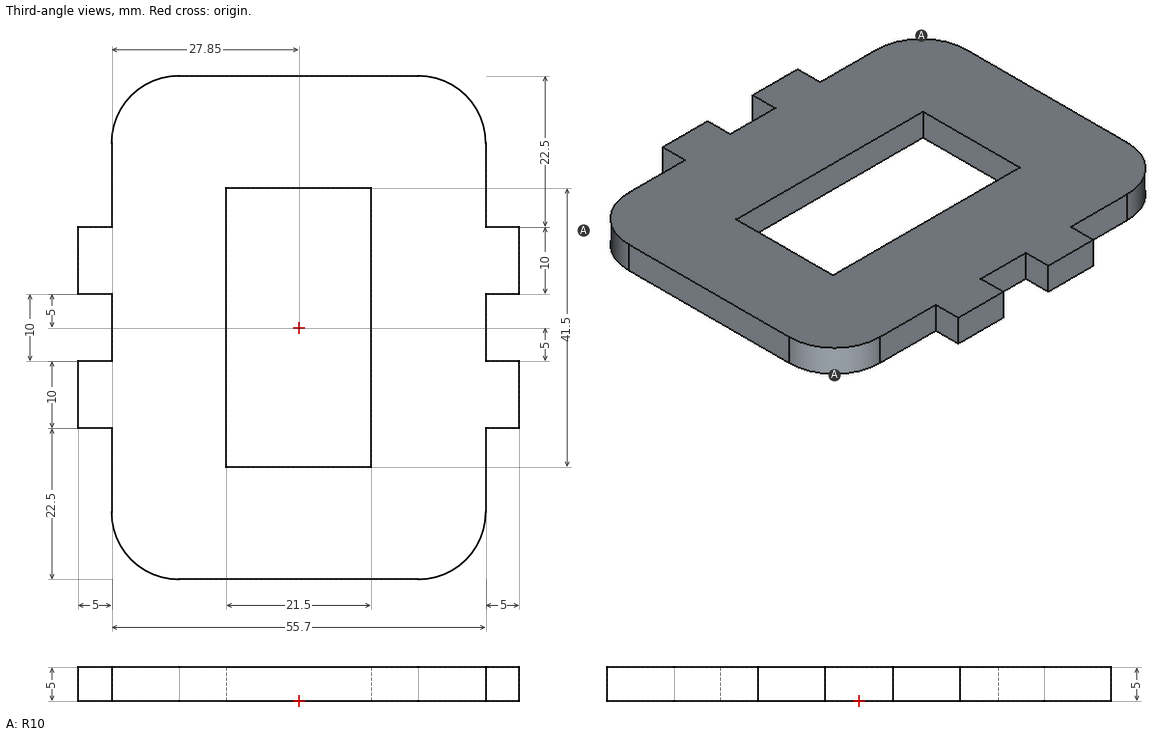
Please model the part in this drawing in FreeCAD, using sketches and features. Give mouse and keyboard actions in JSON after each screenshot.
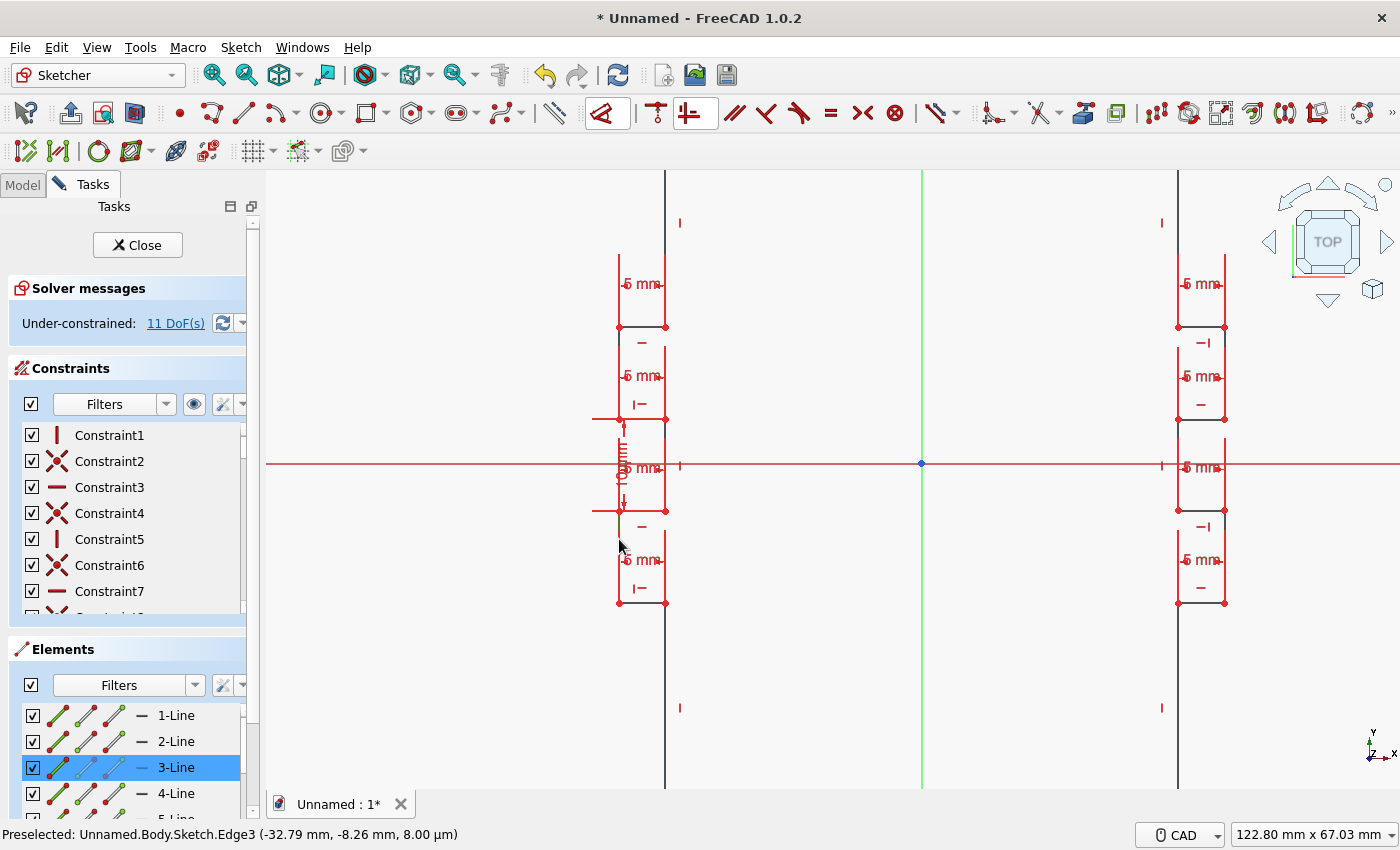
{"action": "key", "text": "i"}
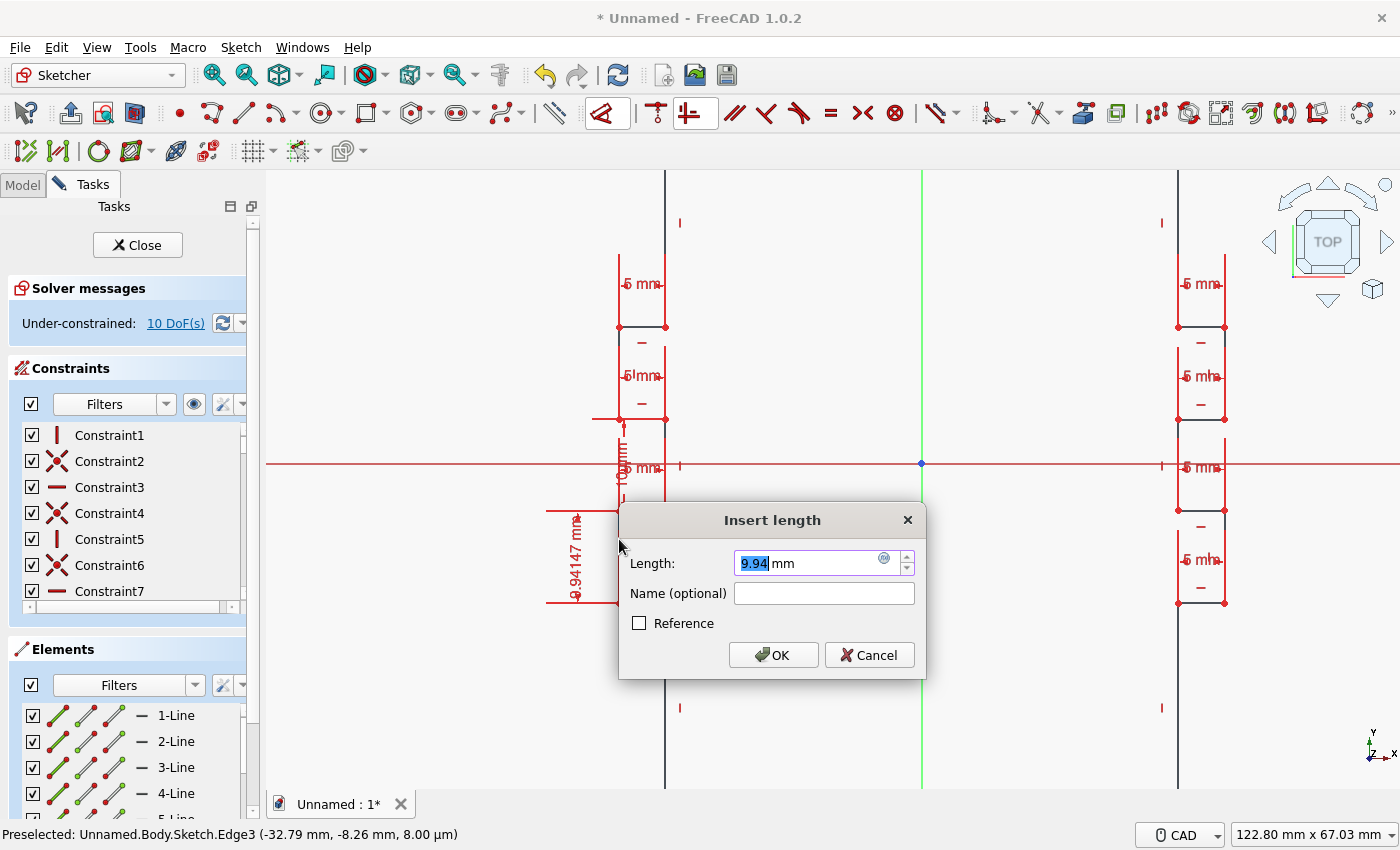
{"action": "type", "text": "10"}
{"action": "key", "text": "Return"}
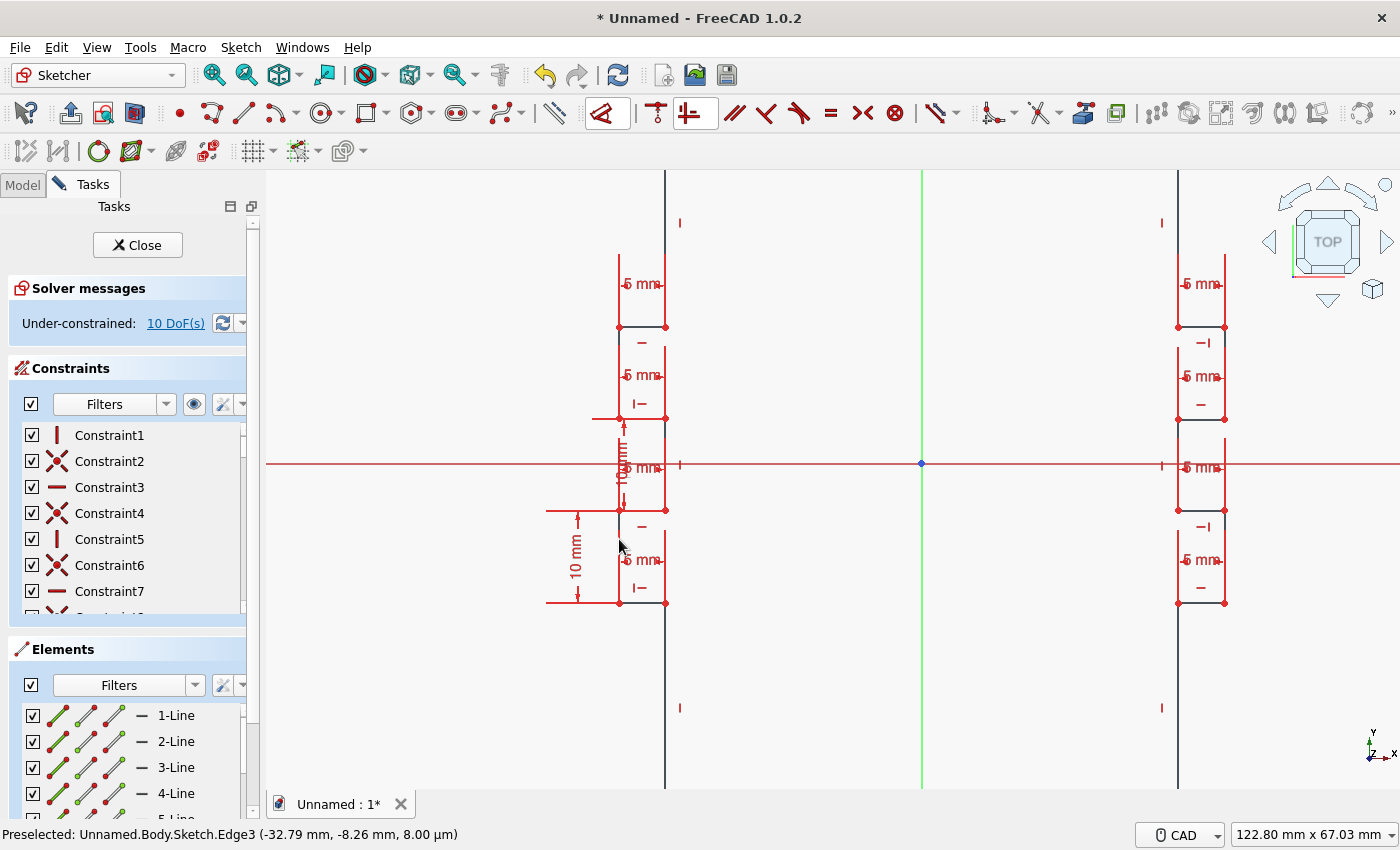
{"action": "left_click", "coordinate": [1225, 575]}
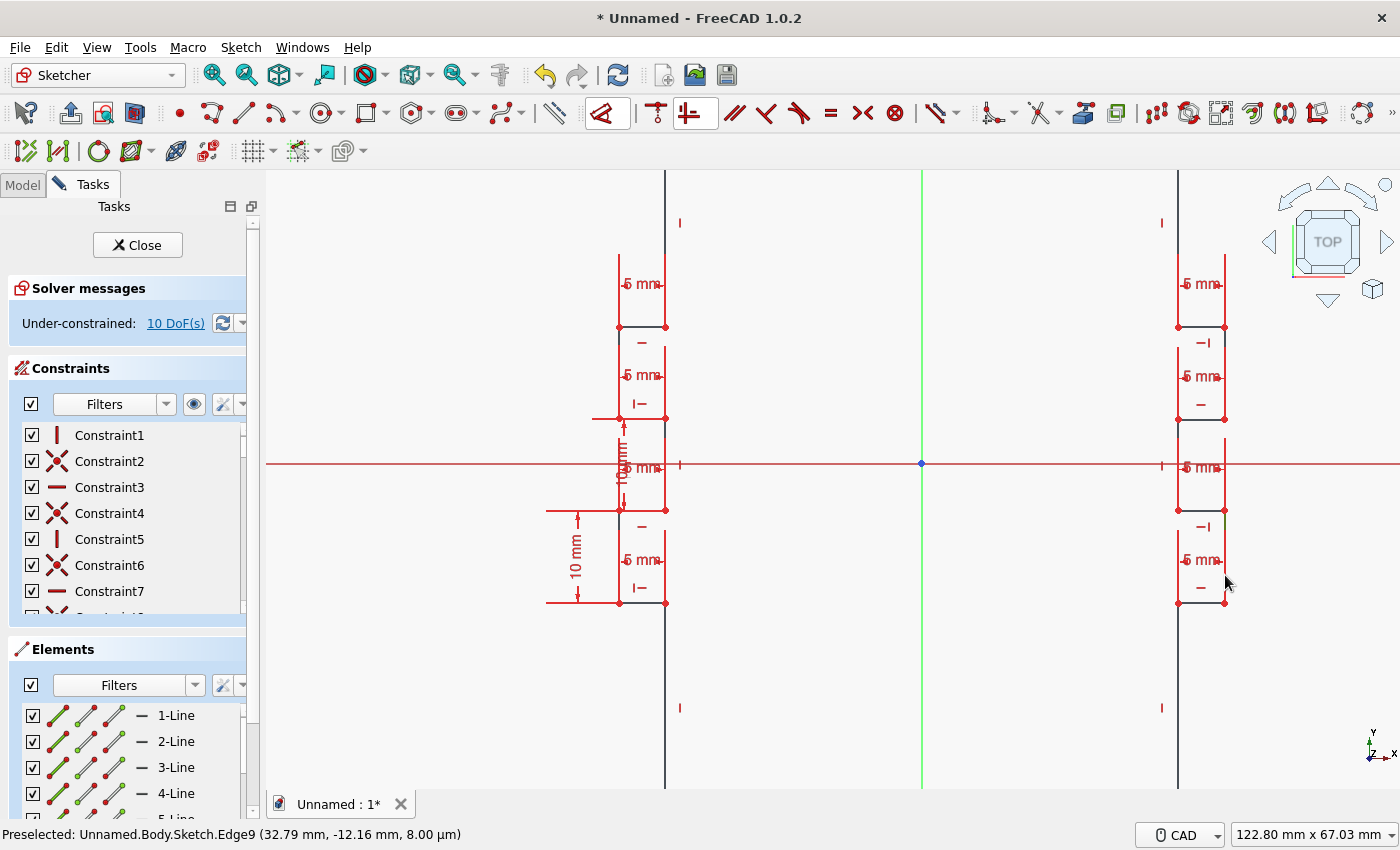
{"action": "key", "text": "i"}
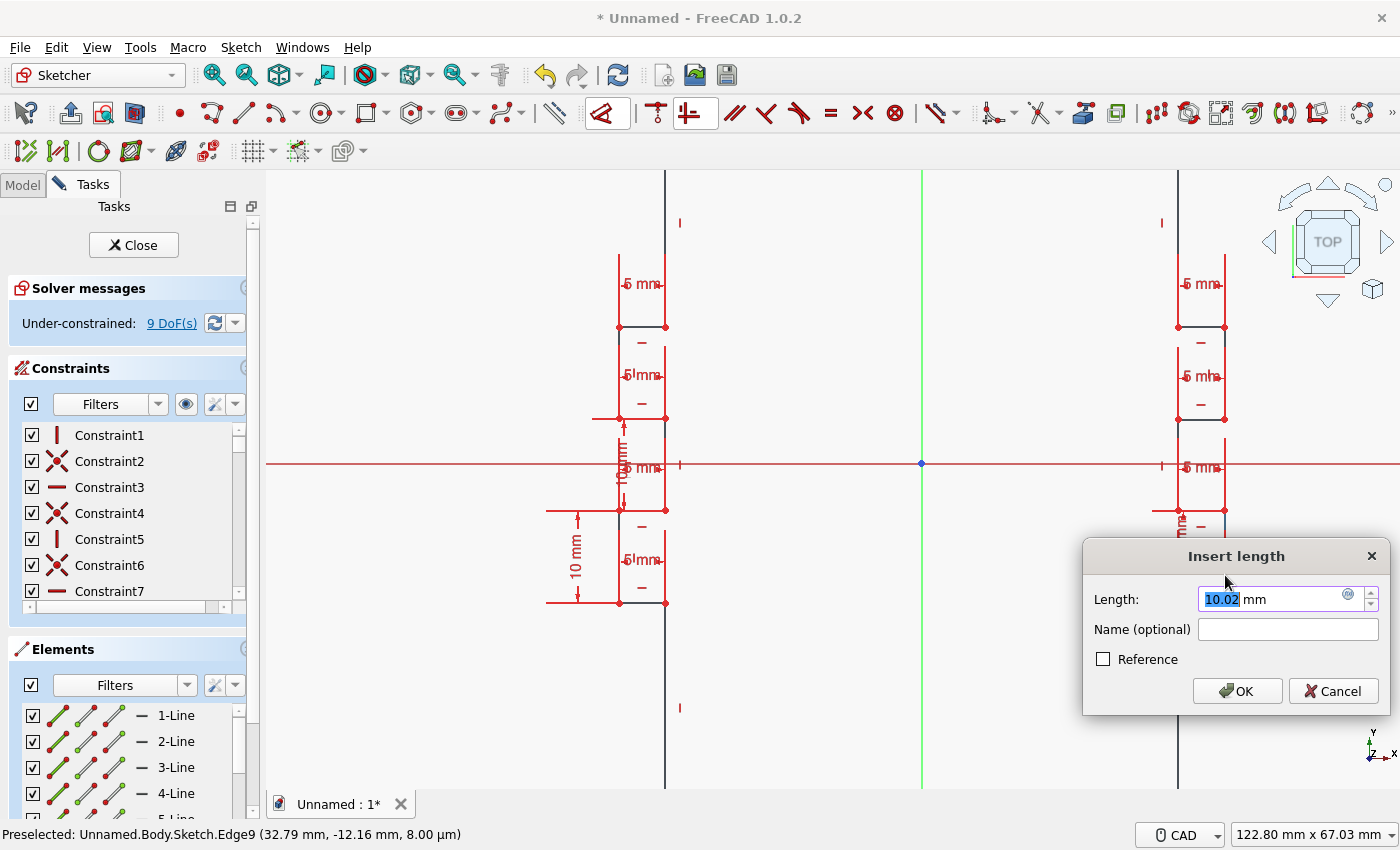
{"action": "type", "text": "10"}
{"action": "key", "text": "Return"}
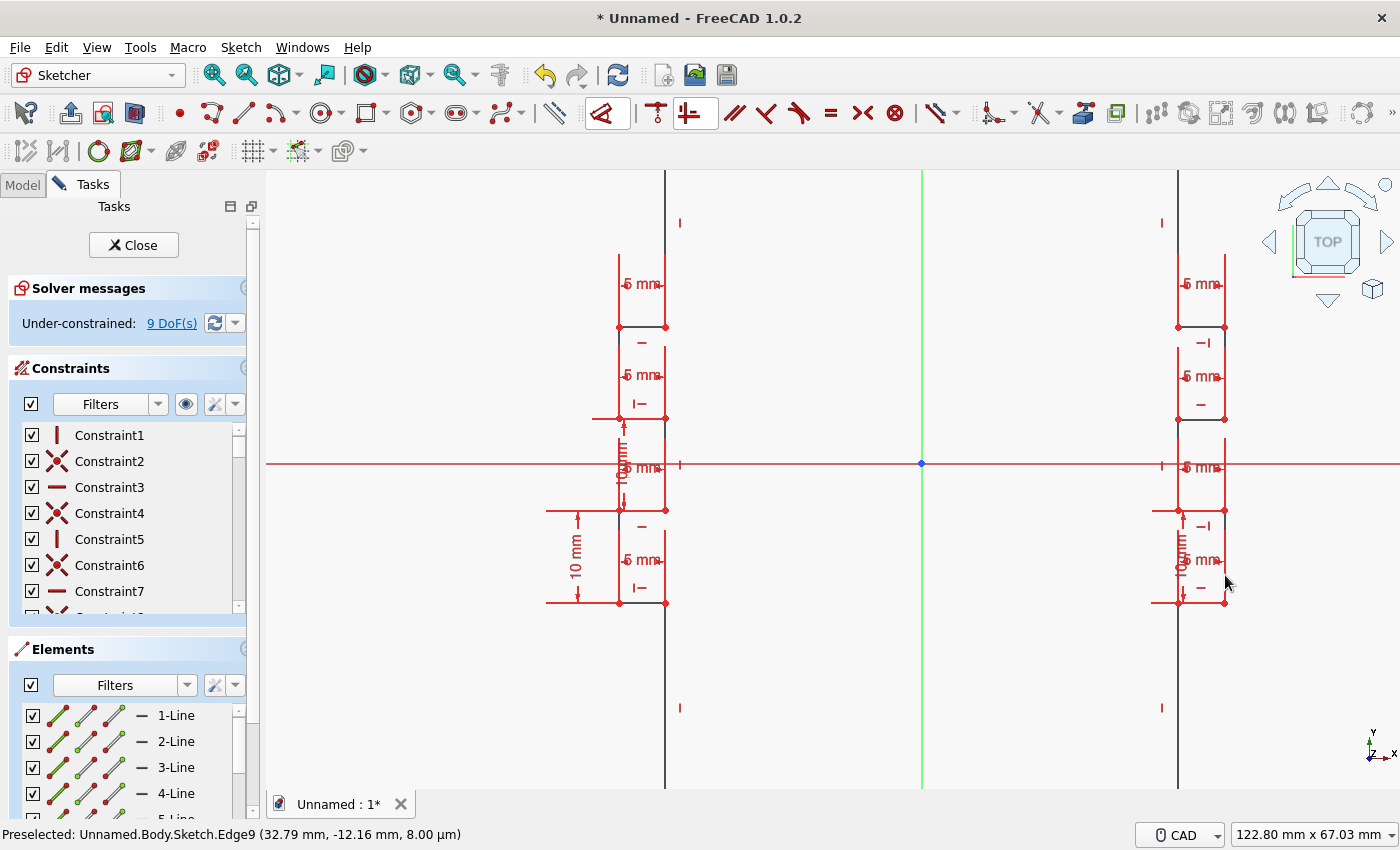
{"action": "left_click", "coordinate": [1178, 483]}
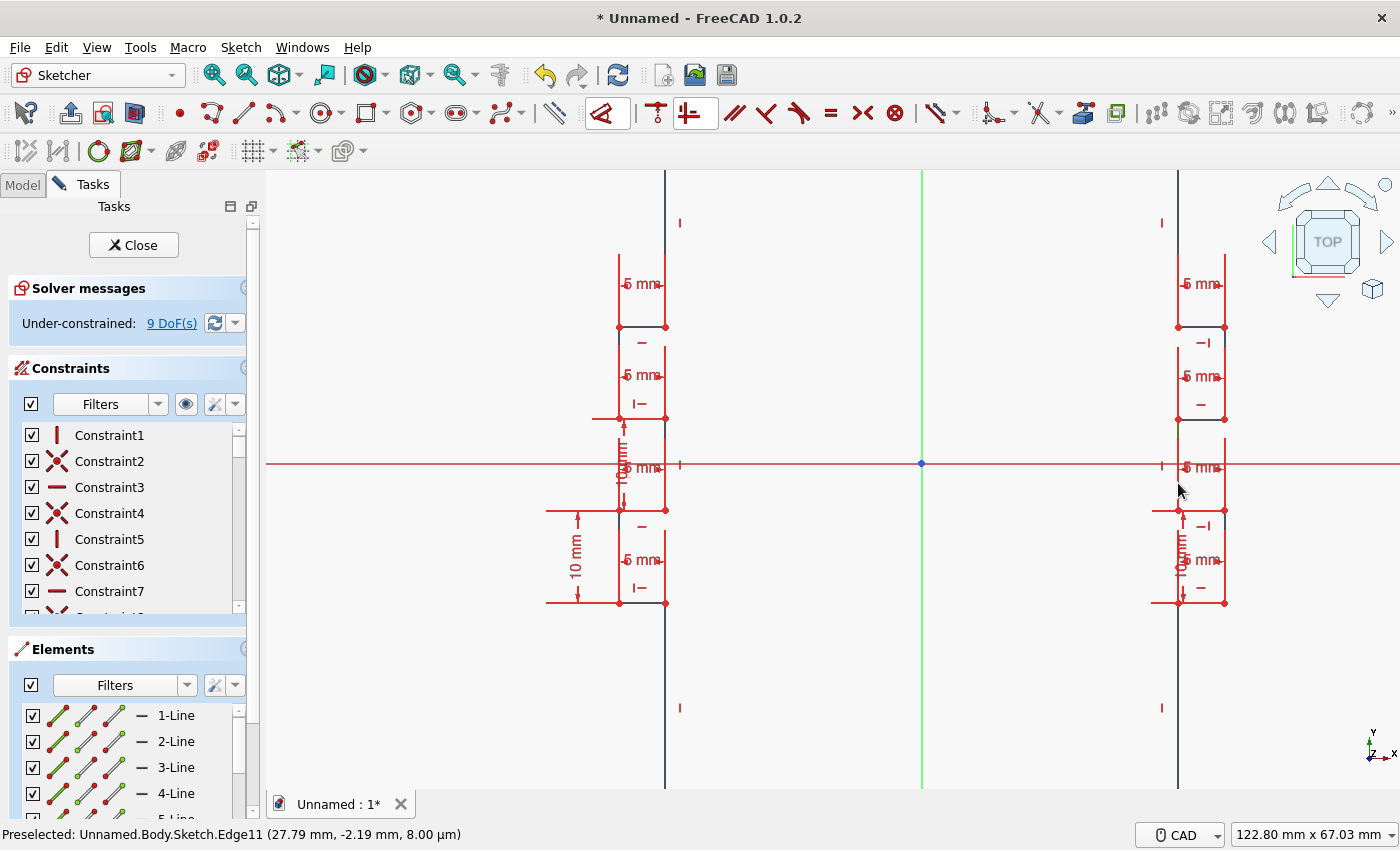
{"action": "key", "text": "i"}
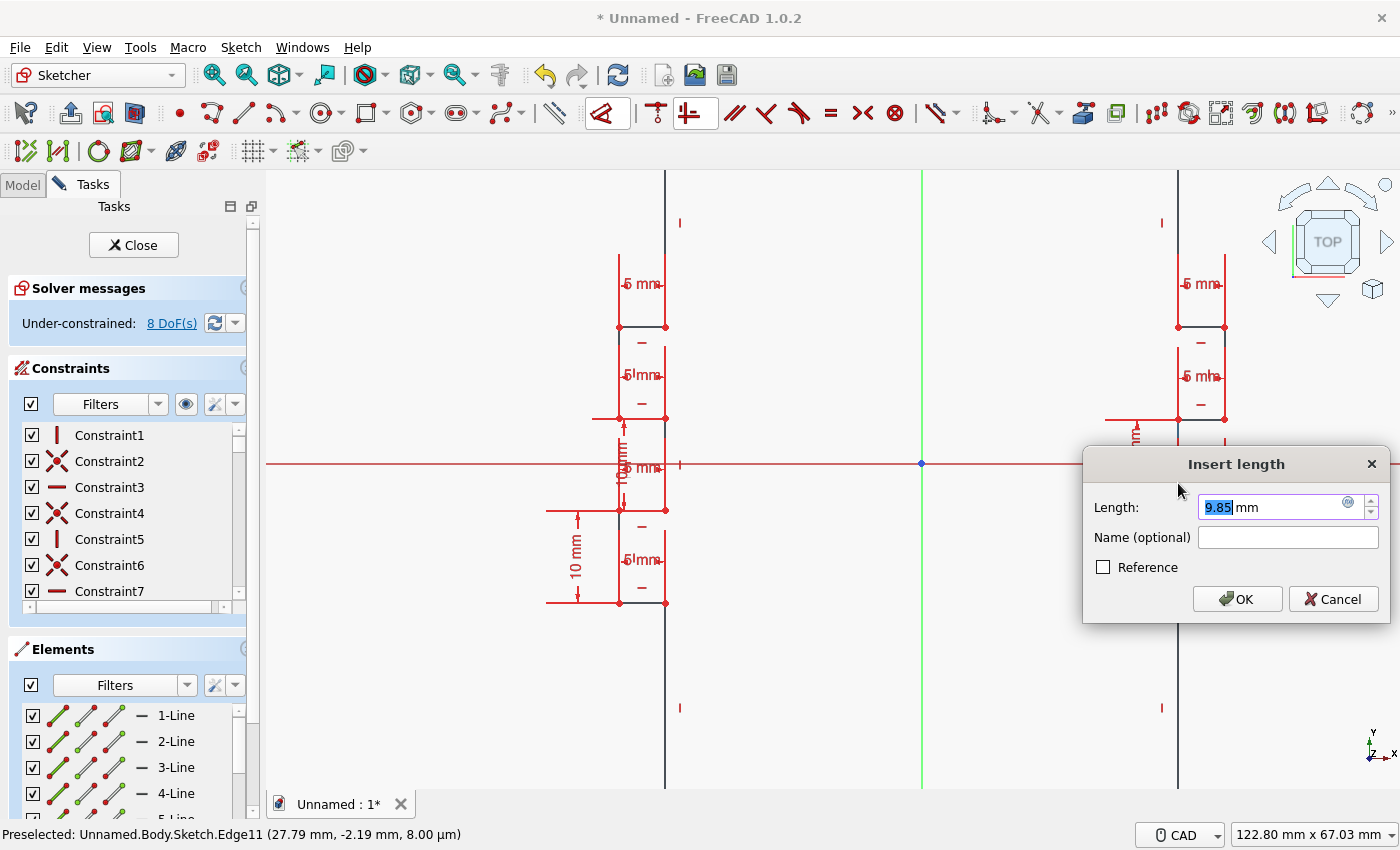
{"action": "type", "text": "10"}
{"action": "key", "text": "Return"}